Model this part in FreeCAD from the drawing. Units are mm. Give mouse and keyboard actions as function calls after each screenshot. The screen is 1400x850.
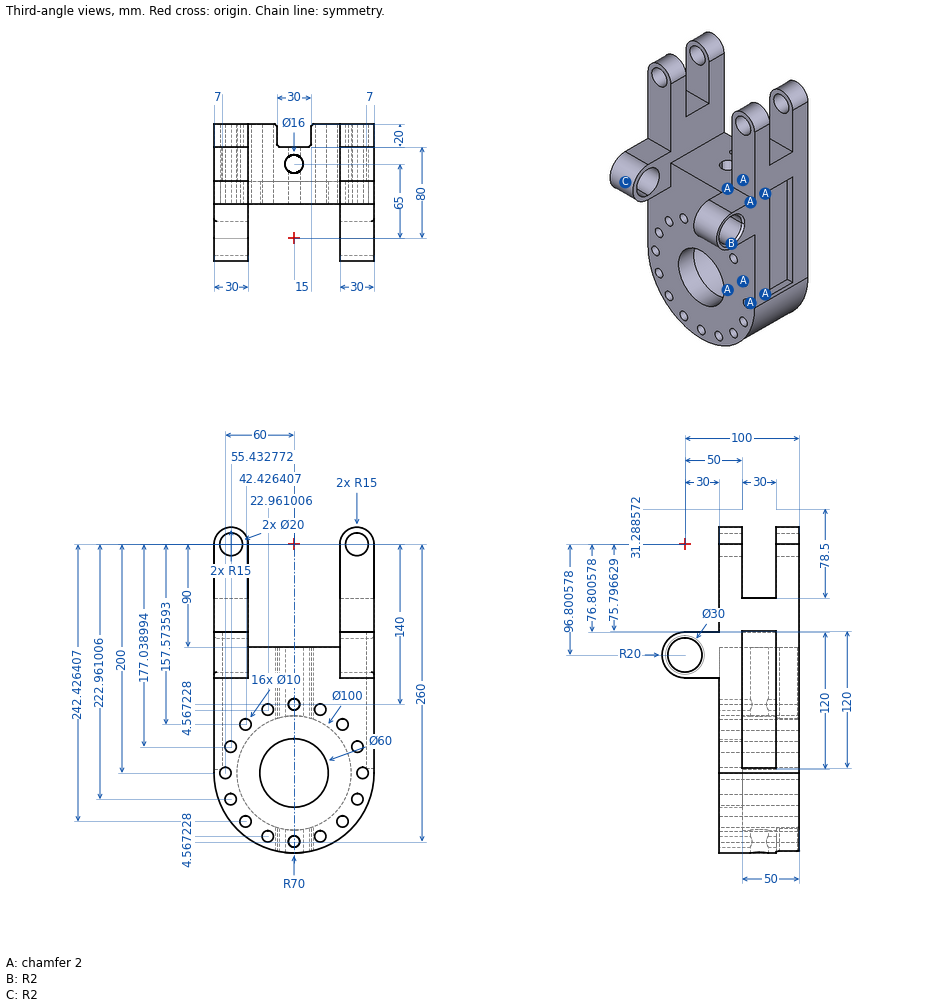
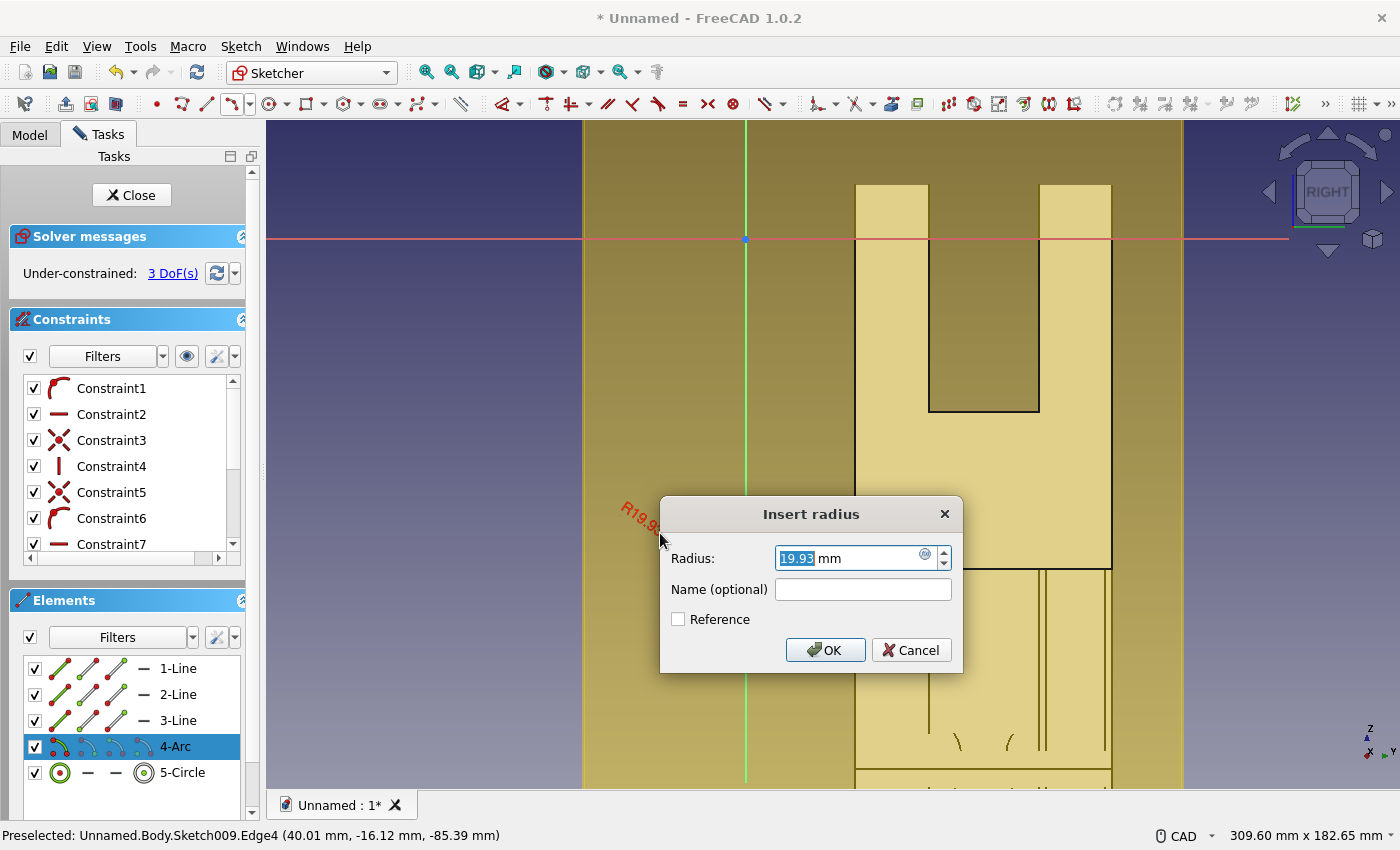
text(20)
key(Return)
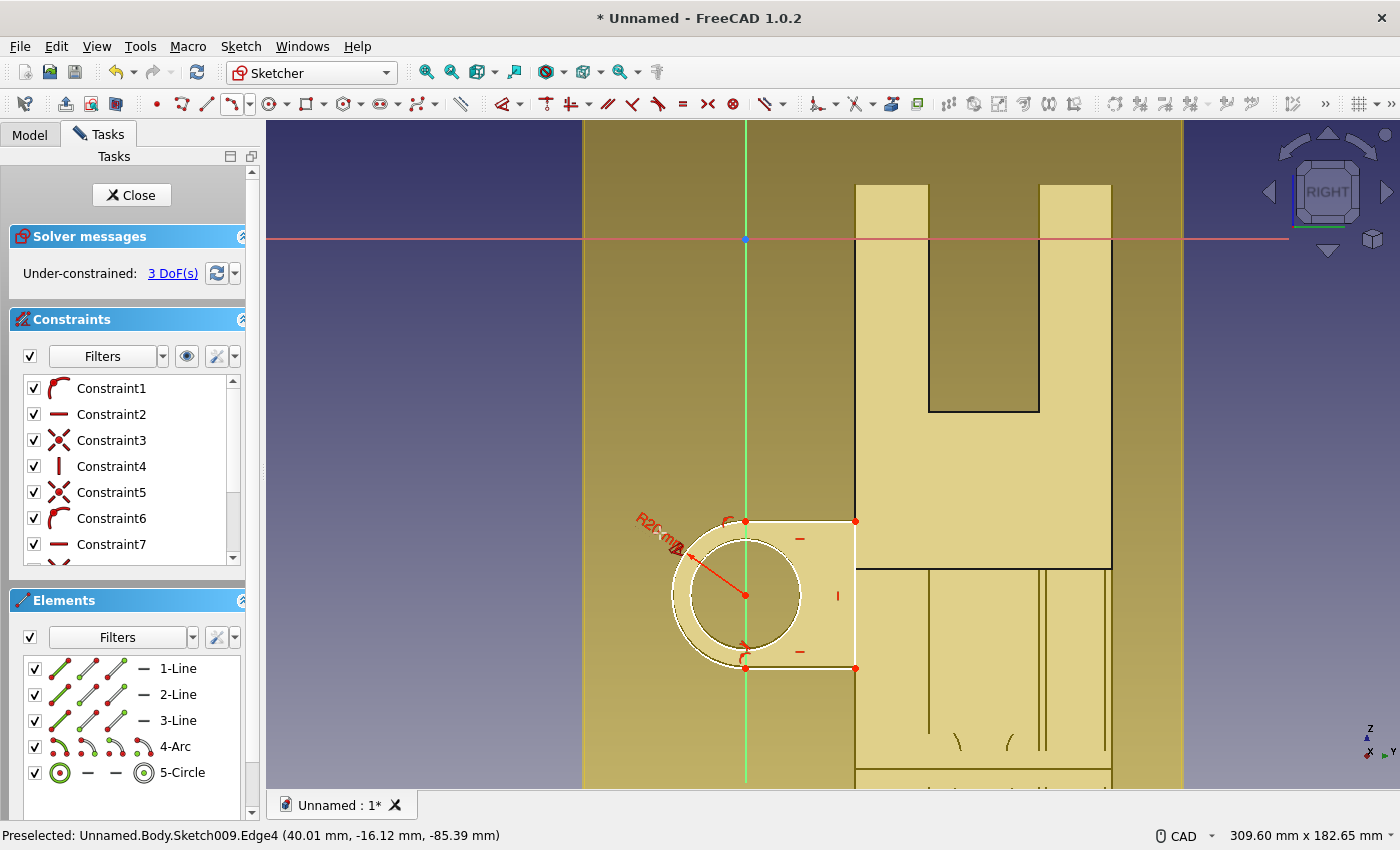
click(784, 556)
click(829, 570)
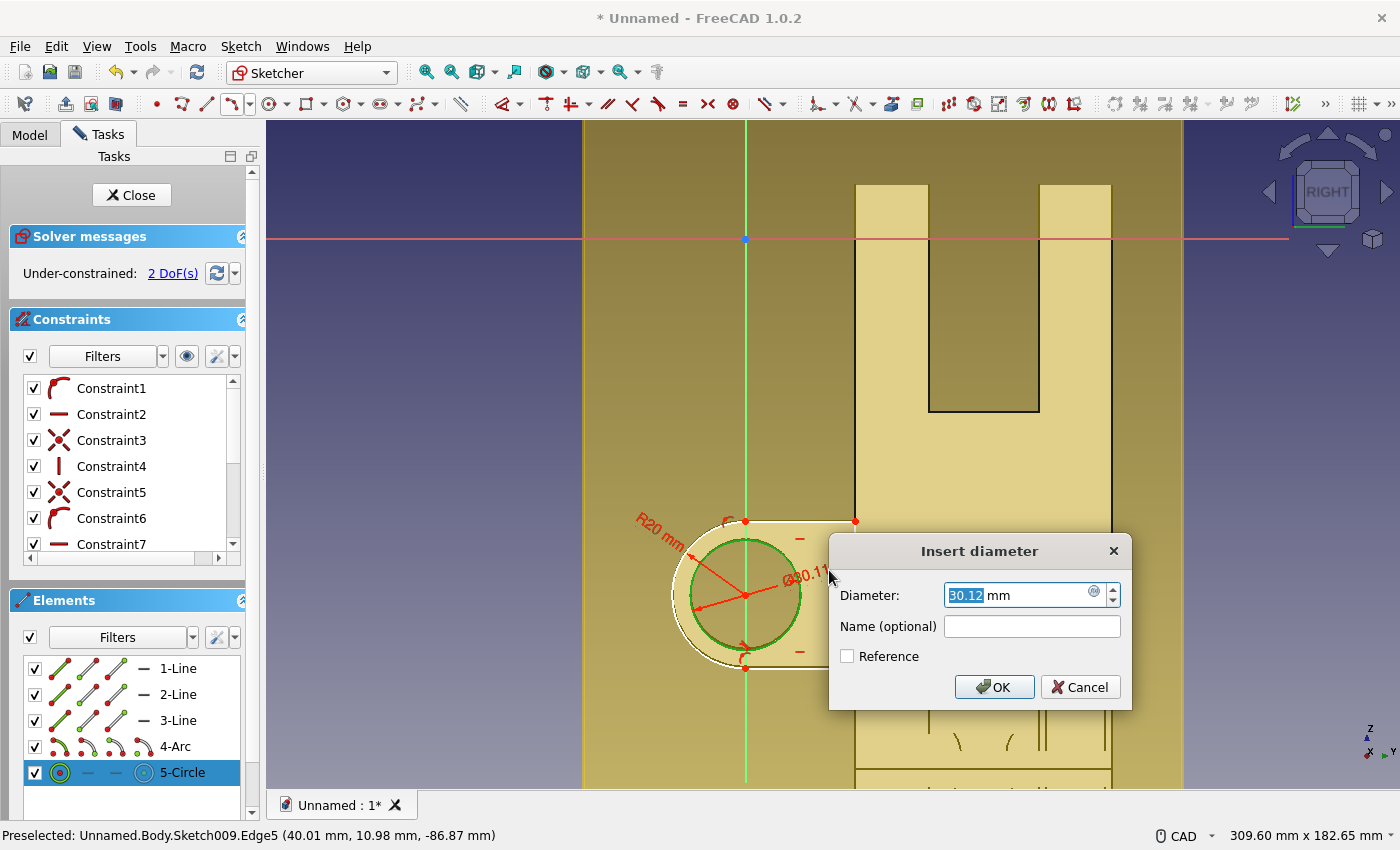
text(30)
key(Return)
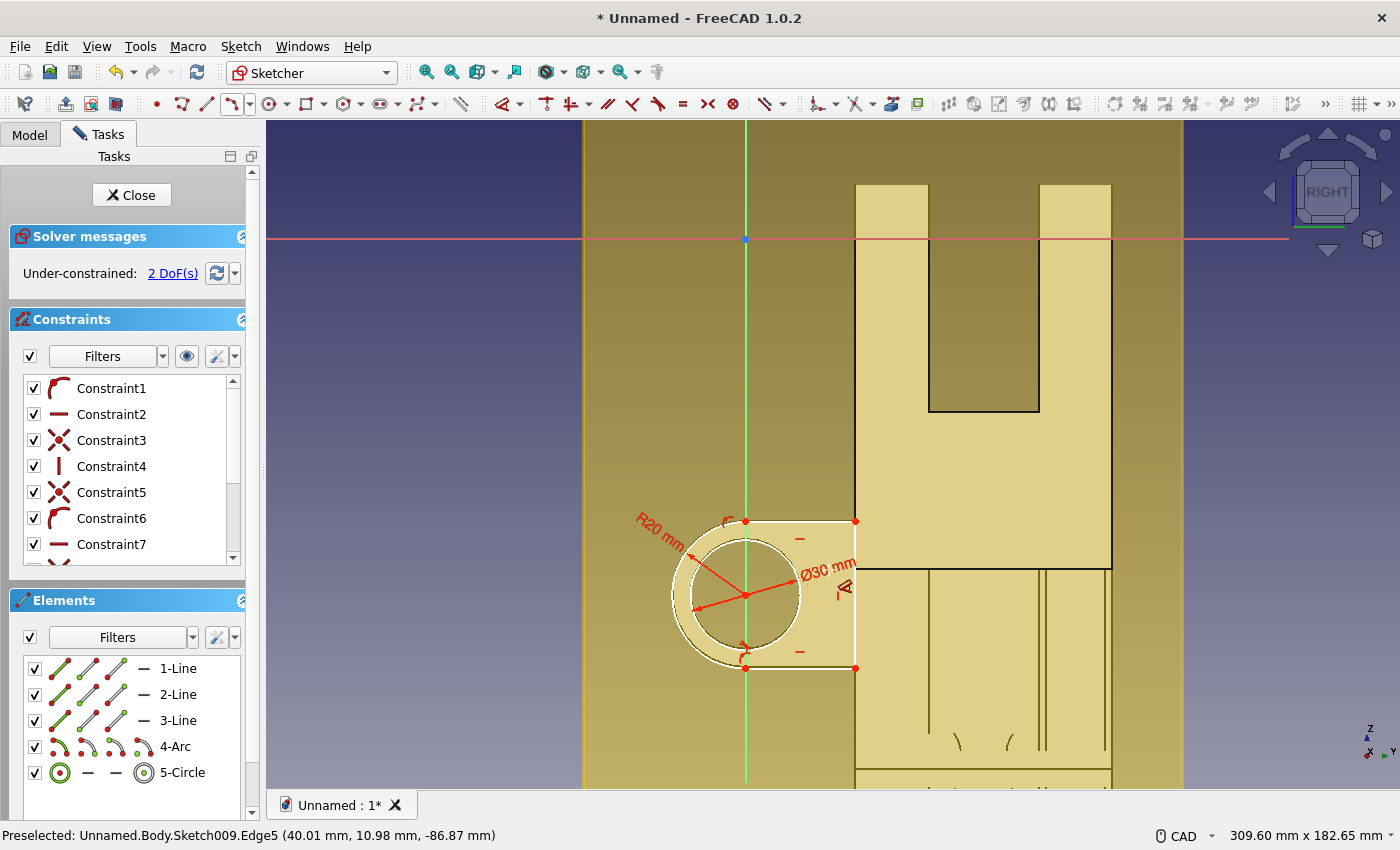
click(778, 669)
click(800, 703)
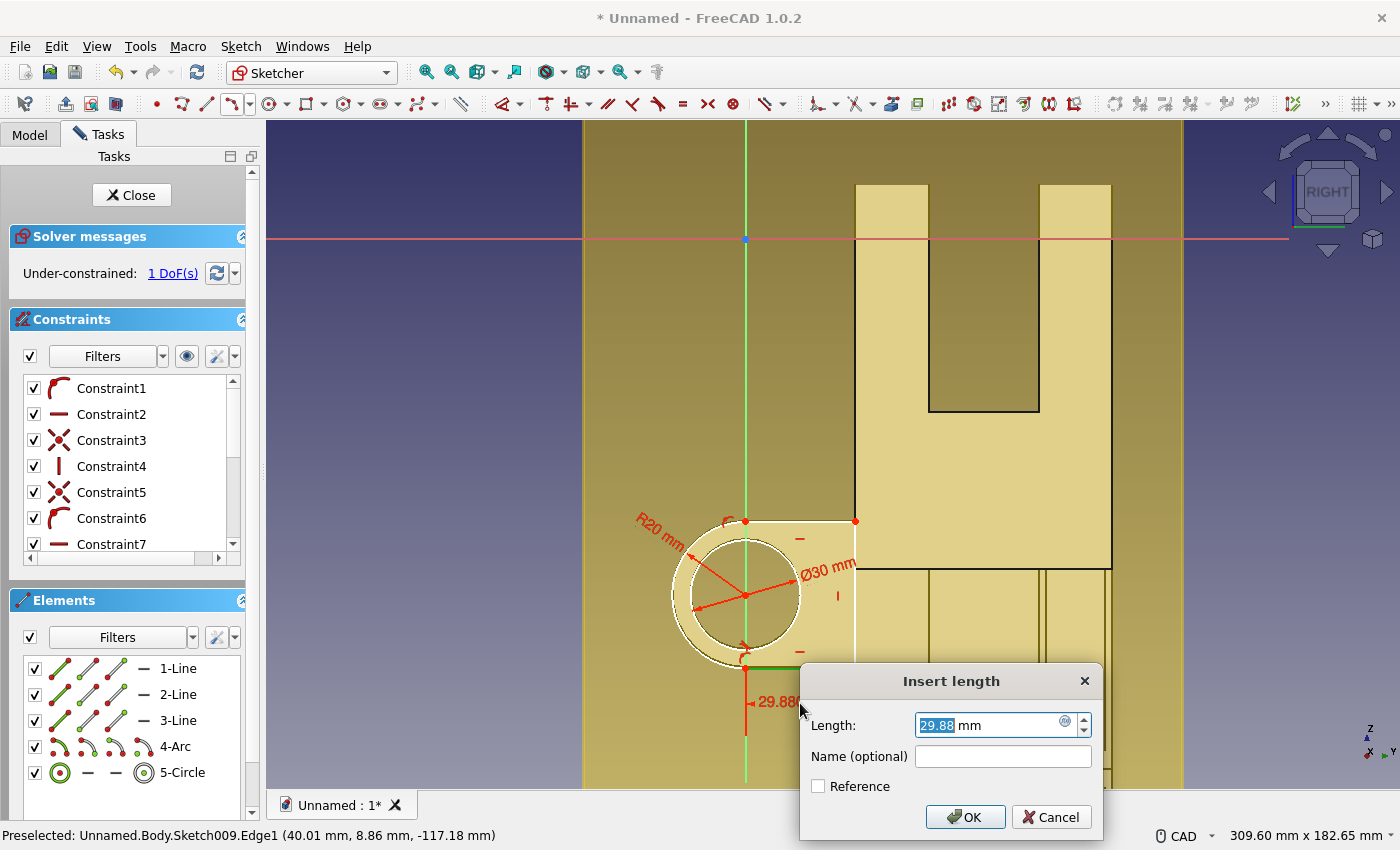
text(30)
key(Return)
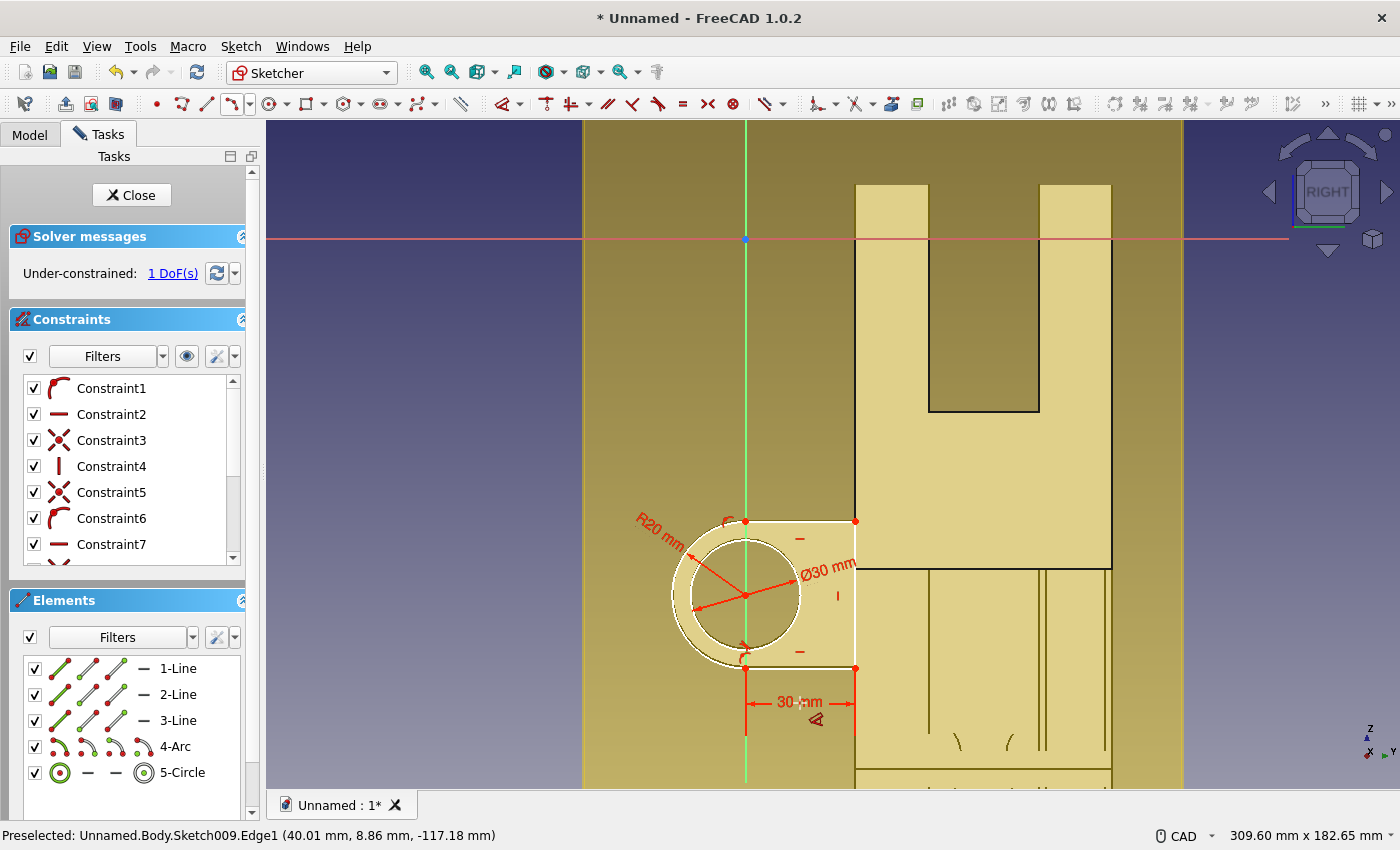
click(746, 595)
click(712, 417)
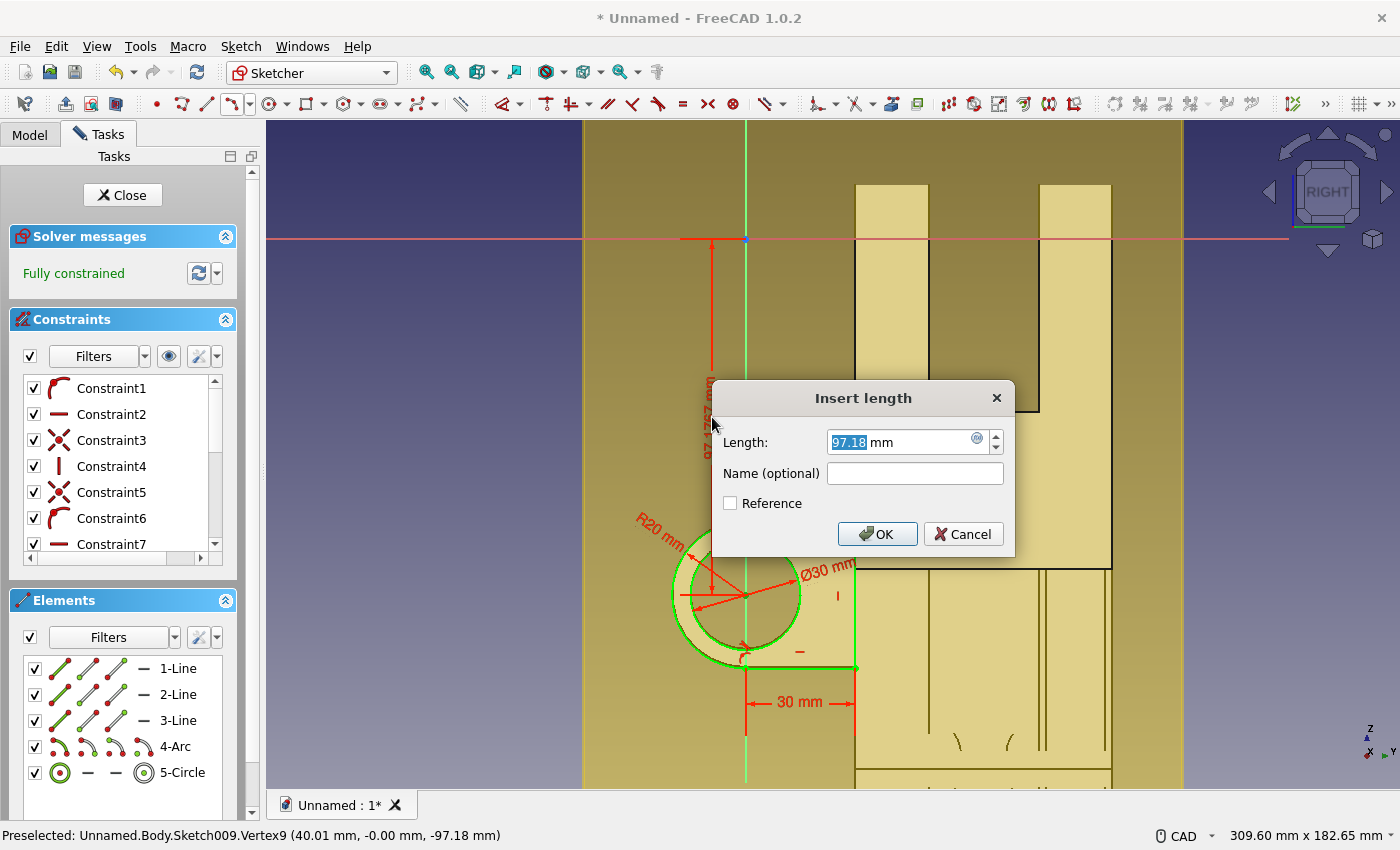
text(96.800578)
key(Return)
key(Escape)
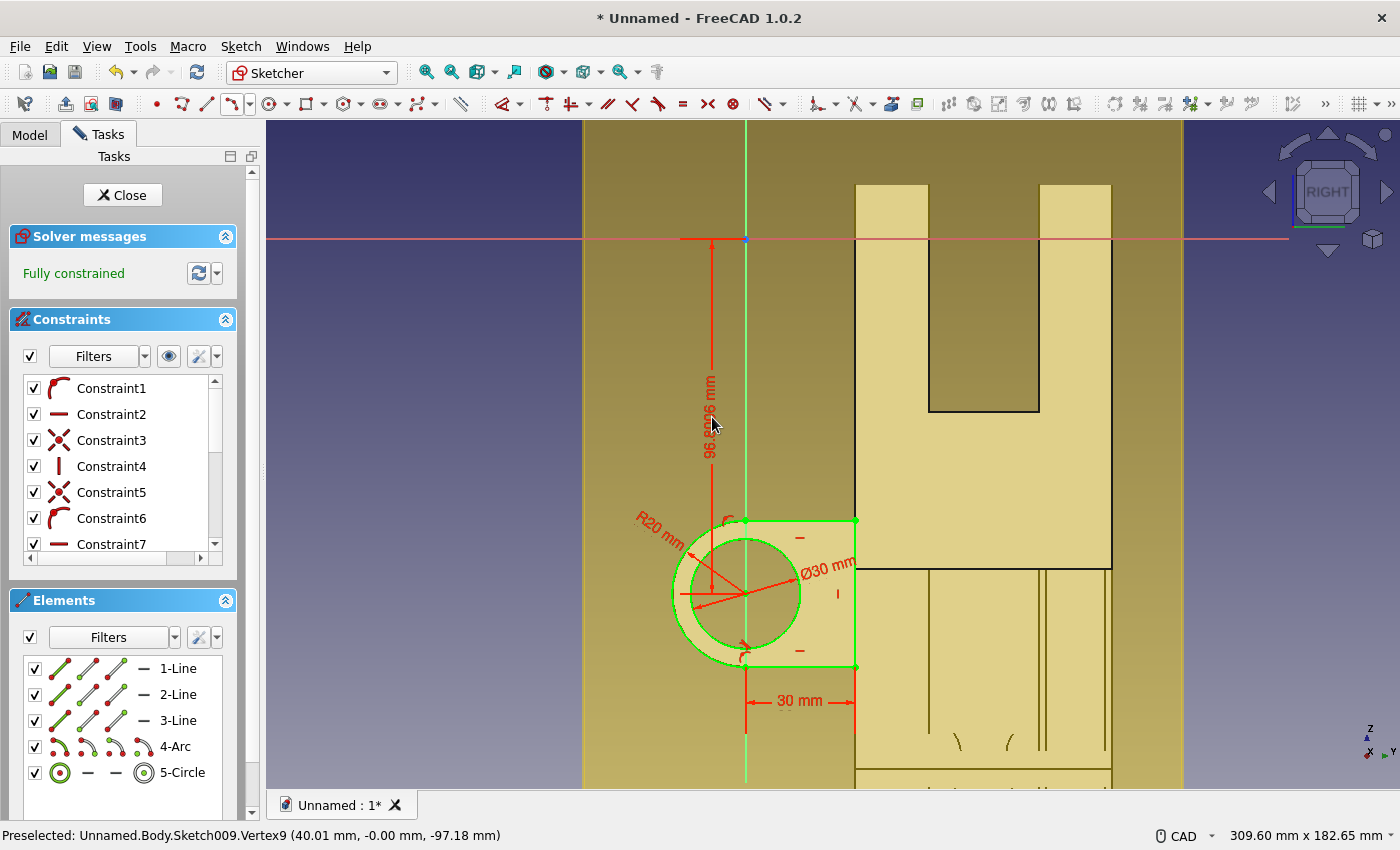
click(123, 195)